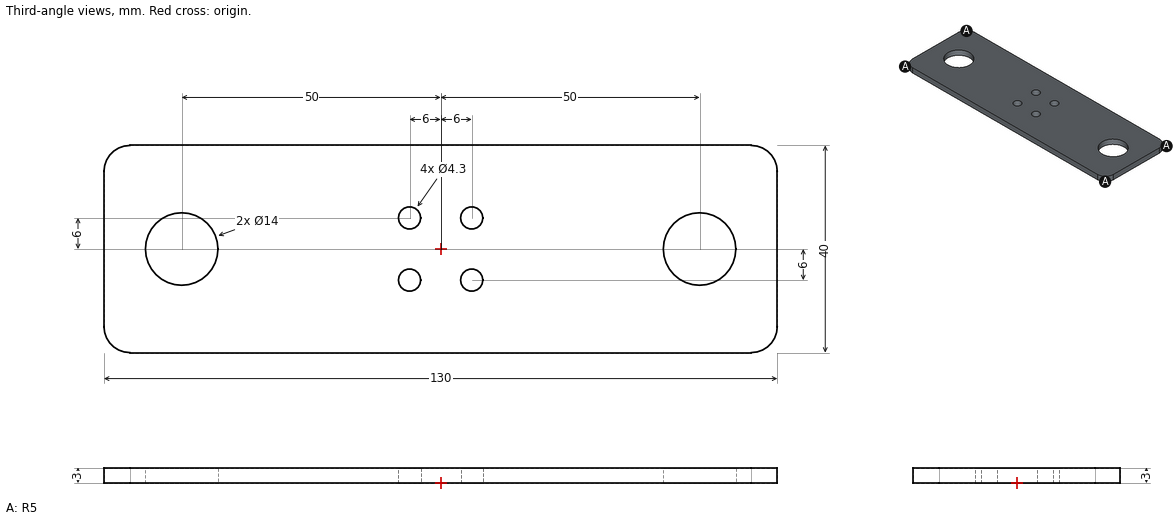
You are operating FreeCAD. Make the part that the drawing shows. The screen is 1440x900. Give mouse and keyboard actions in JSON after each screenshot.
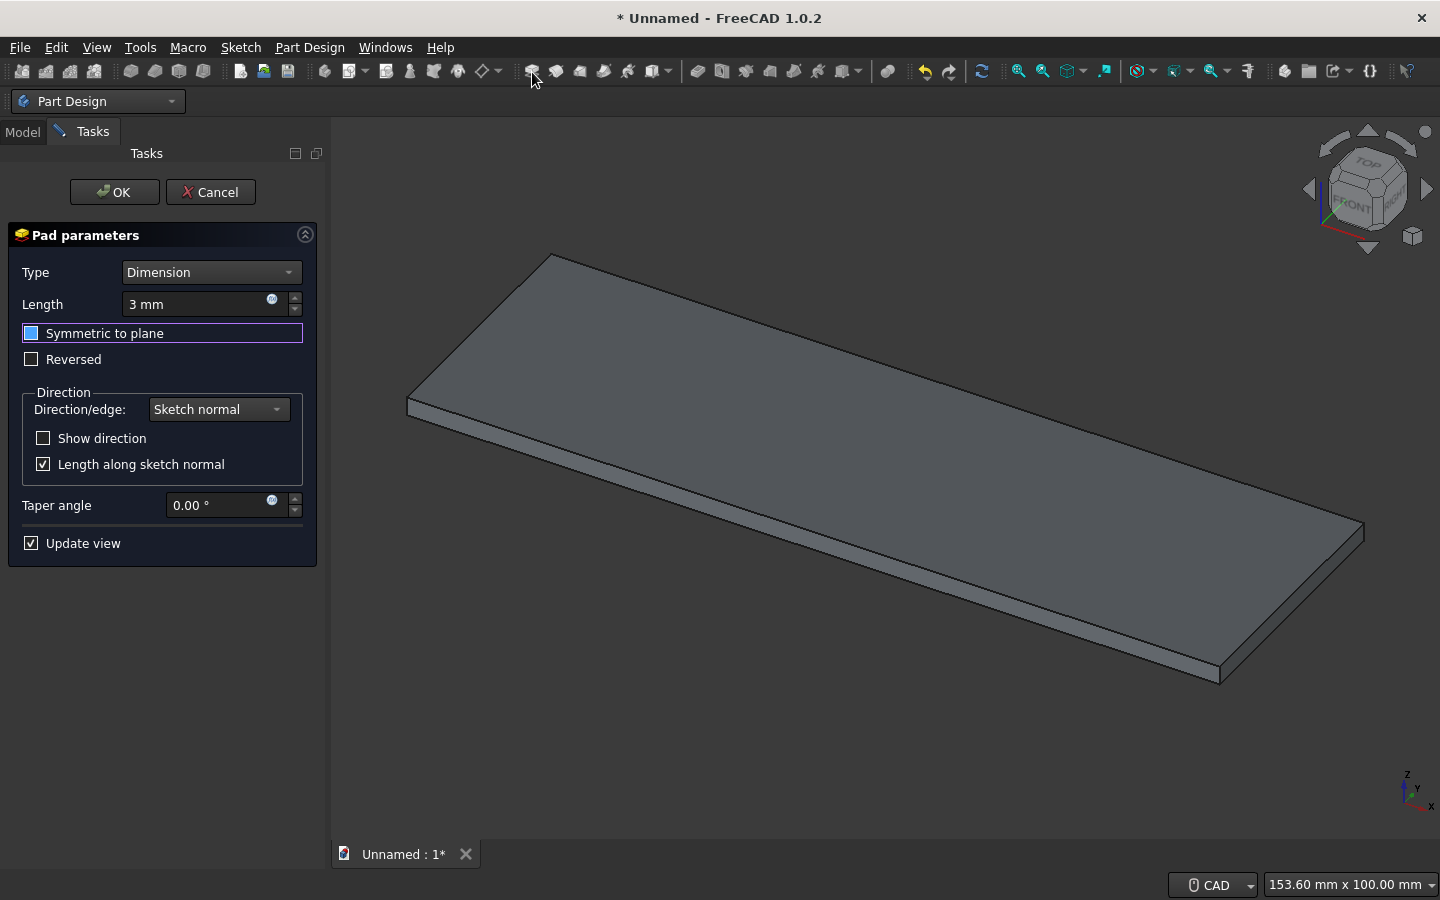
{"action": "left_click", "coordinate": [115, 192]}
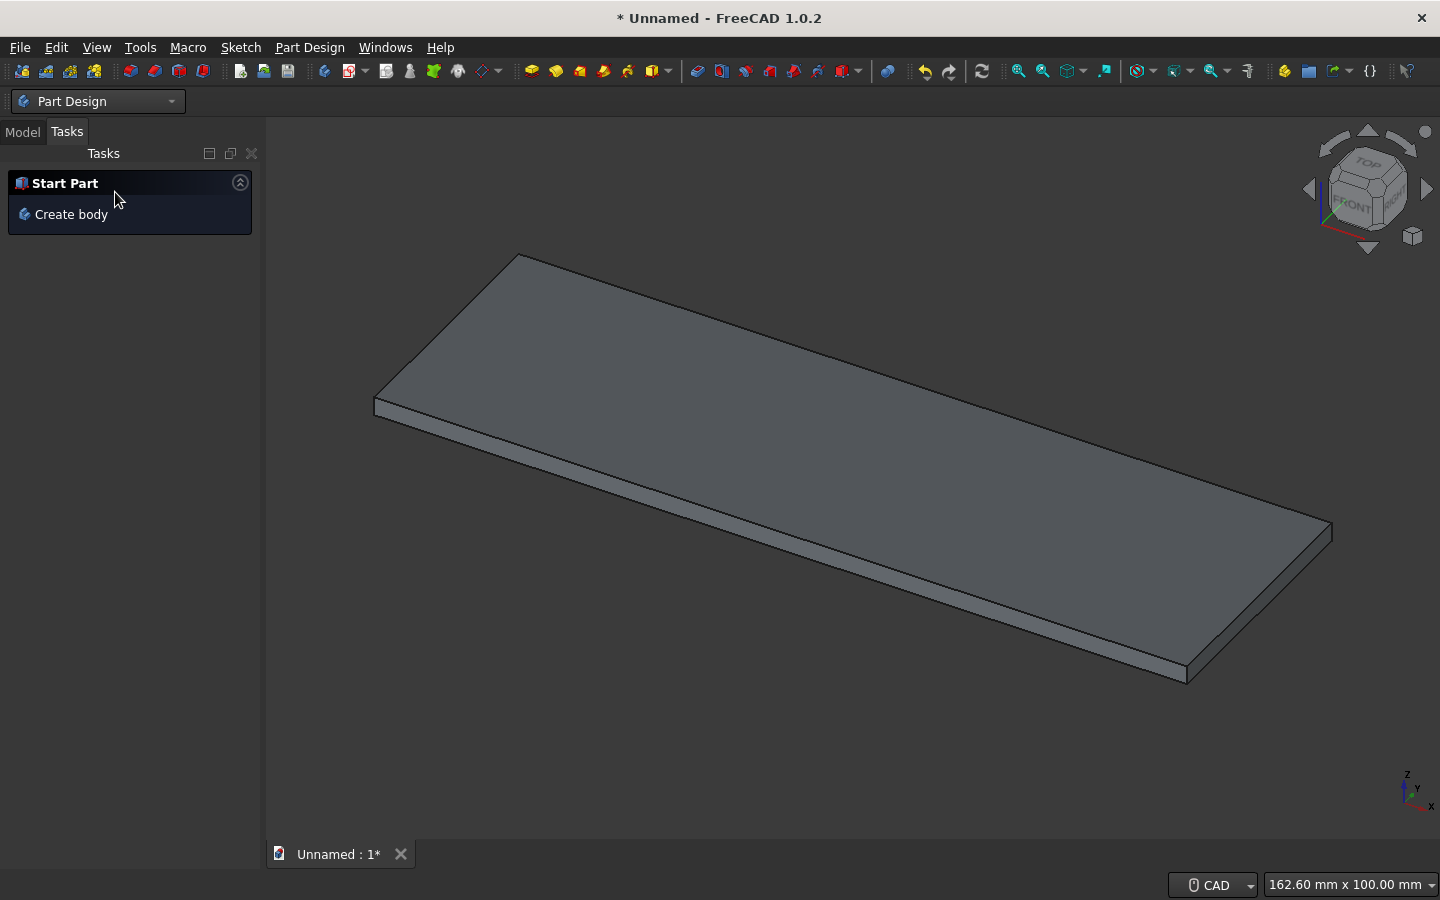
{"action": "left_click", "coordinate": [1085, 536]}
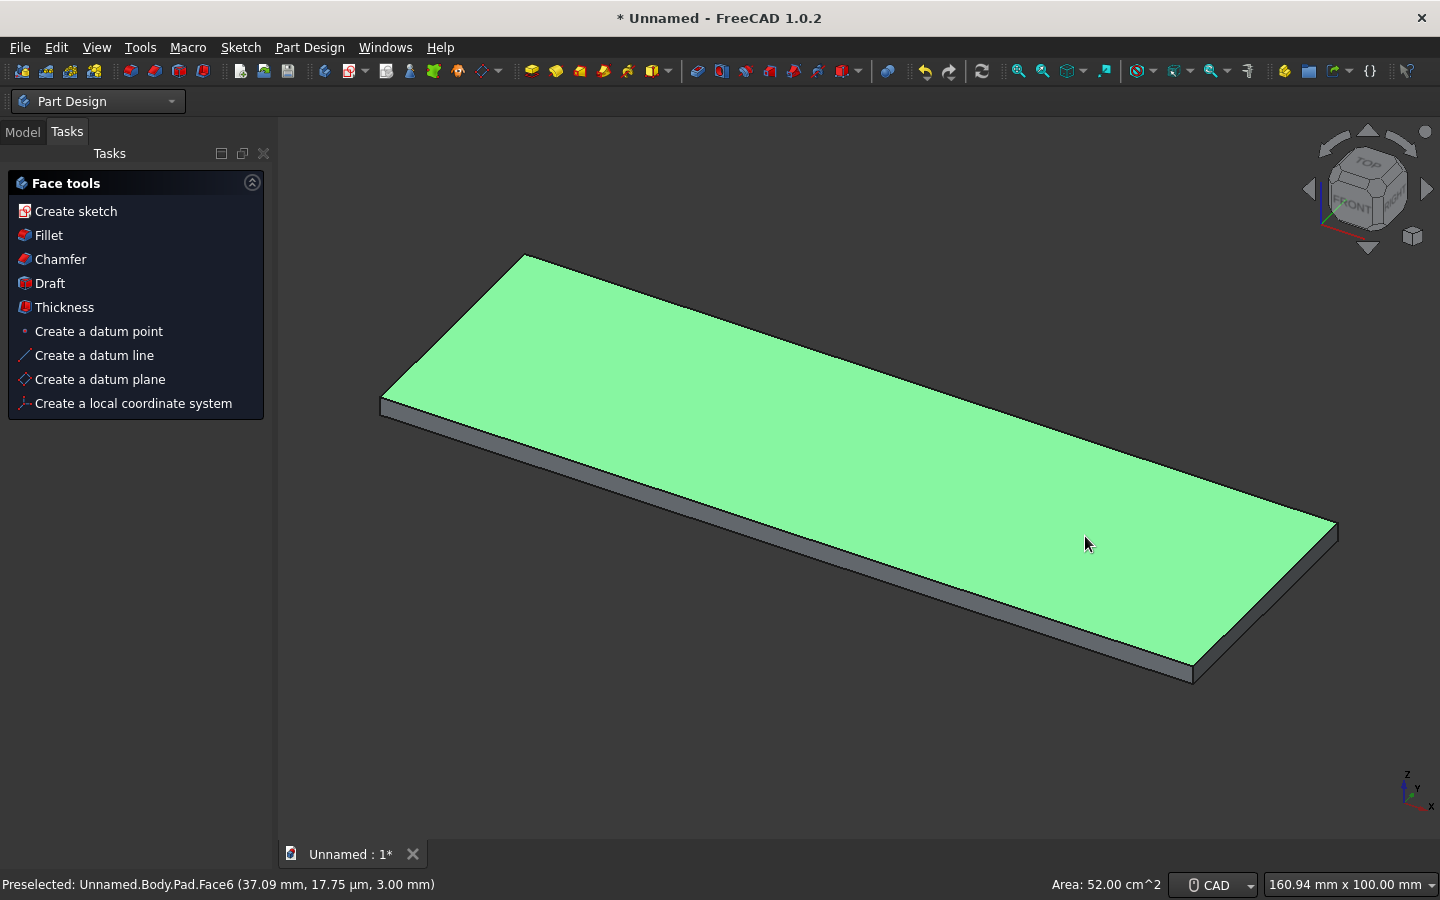
{"action": "left_click", "coordinate": [350, 72]}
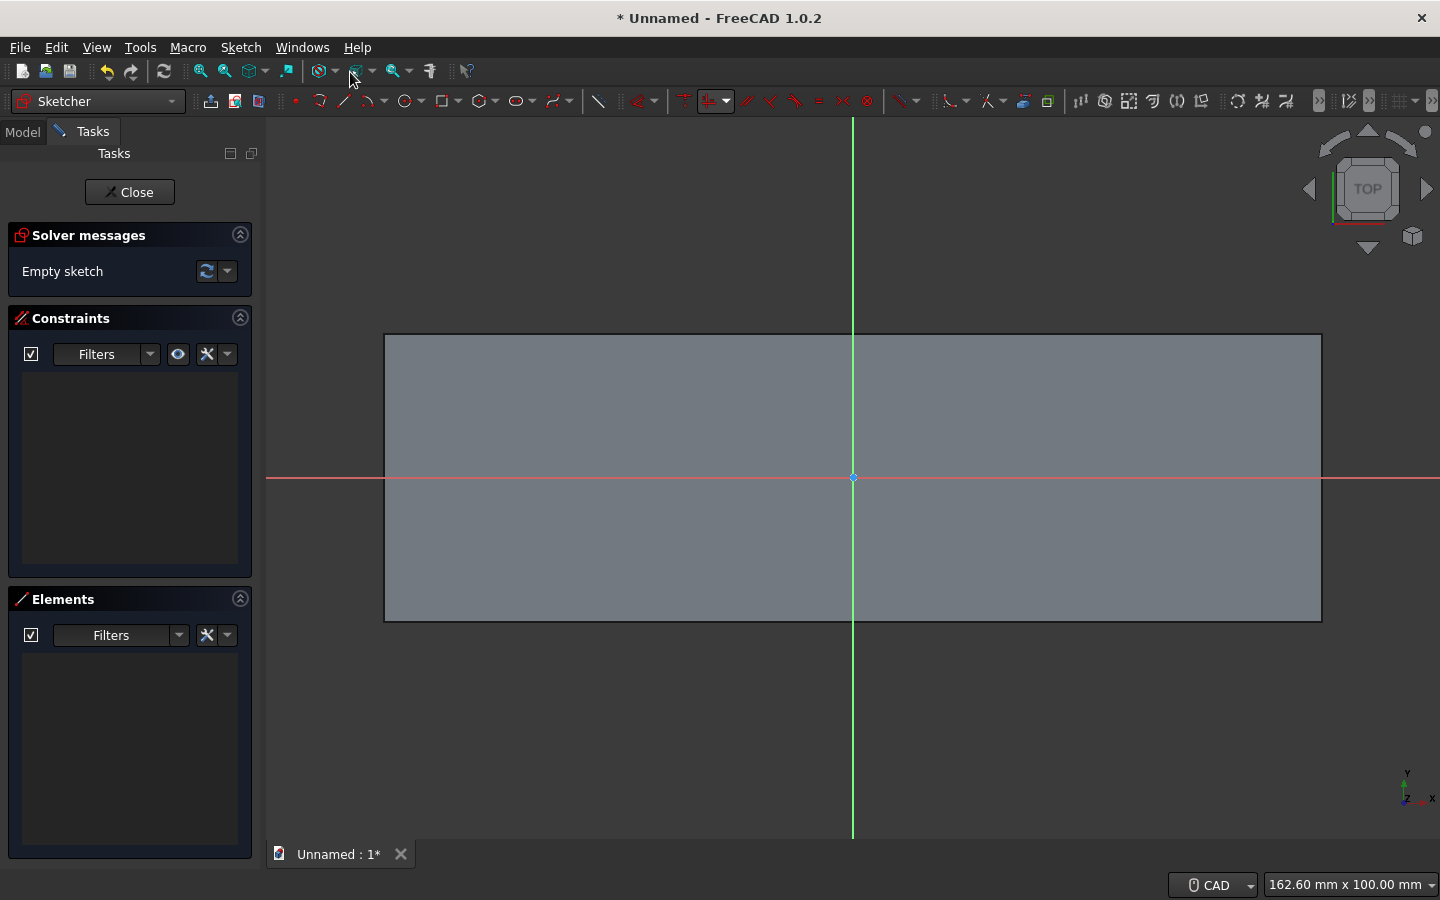
{"action": "scroll", "coordinate": [475, 478], "scroll_direction": "down", "scroll_amount": 1}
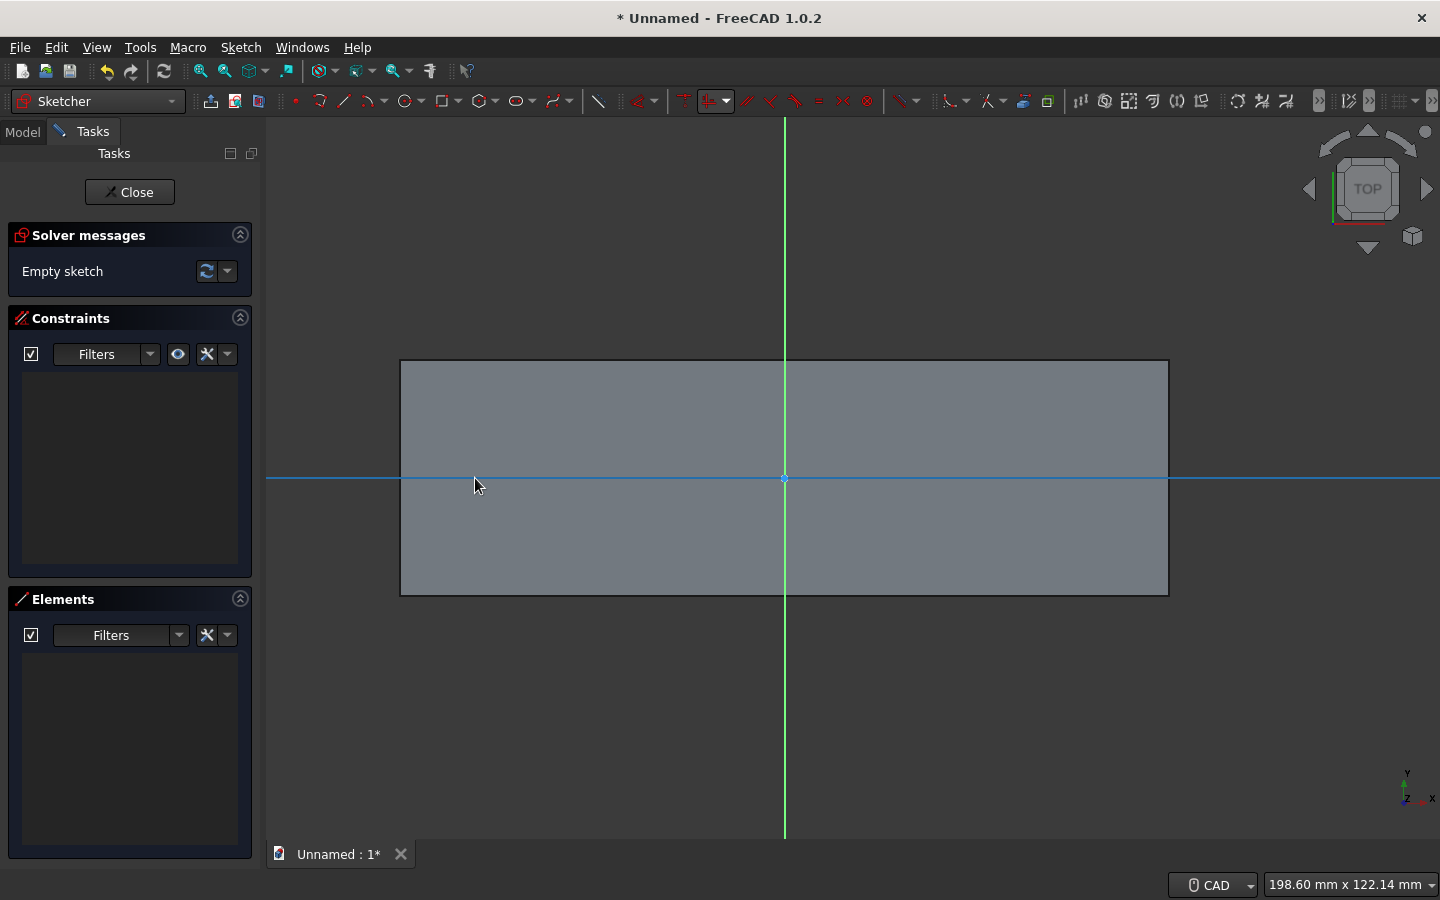
{"action": "key", "text": "g c"}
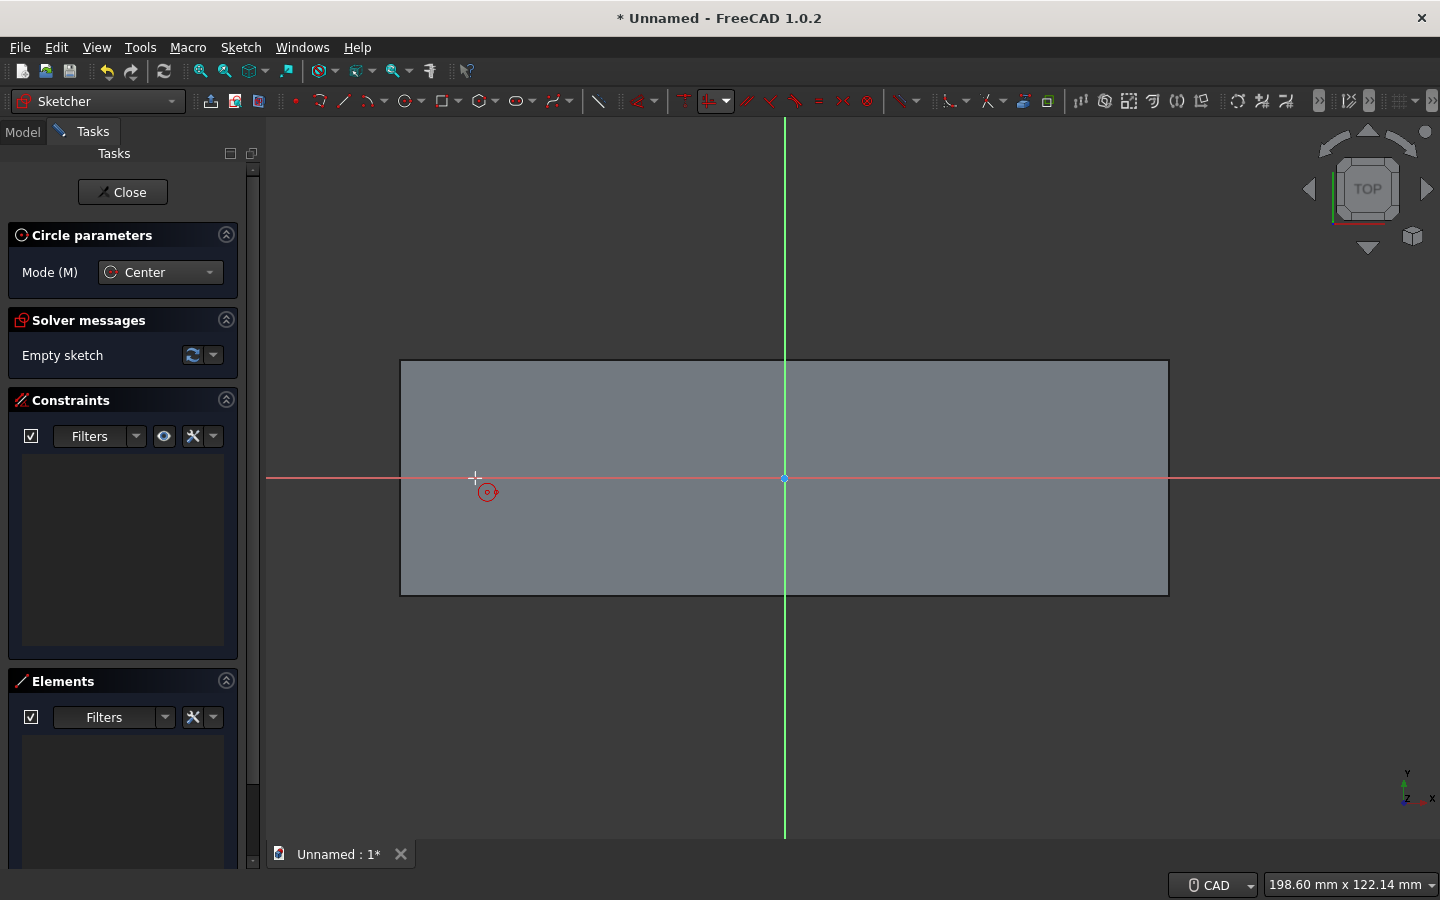
{"action": "left_click", "coordinate": [489, 478]}
{"action": "left_click", "coordinate": [518, 449]}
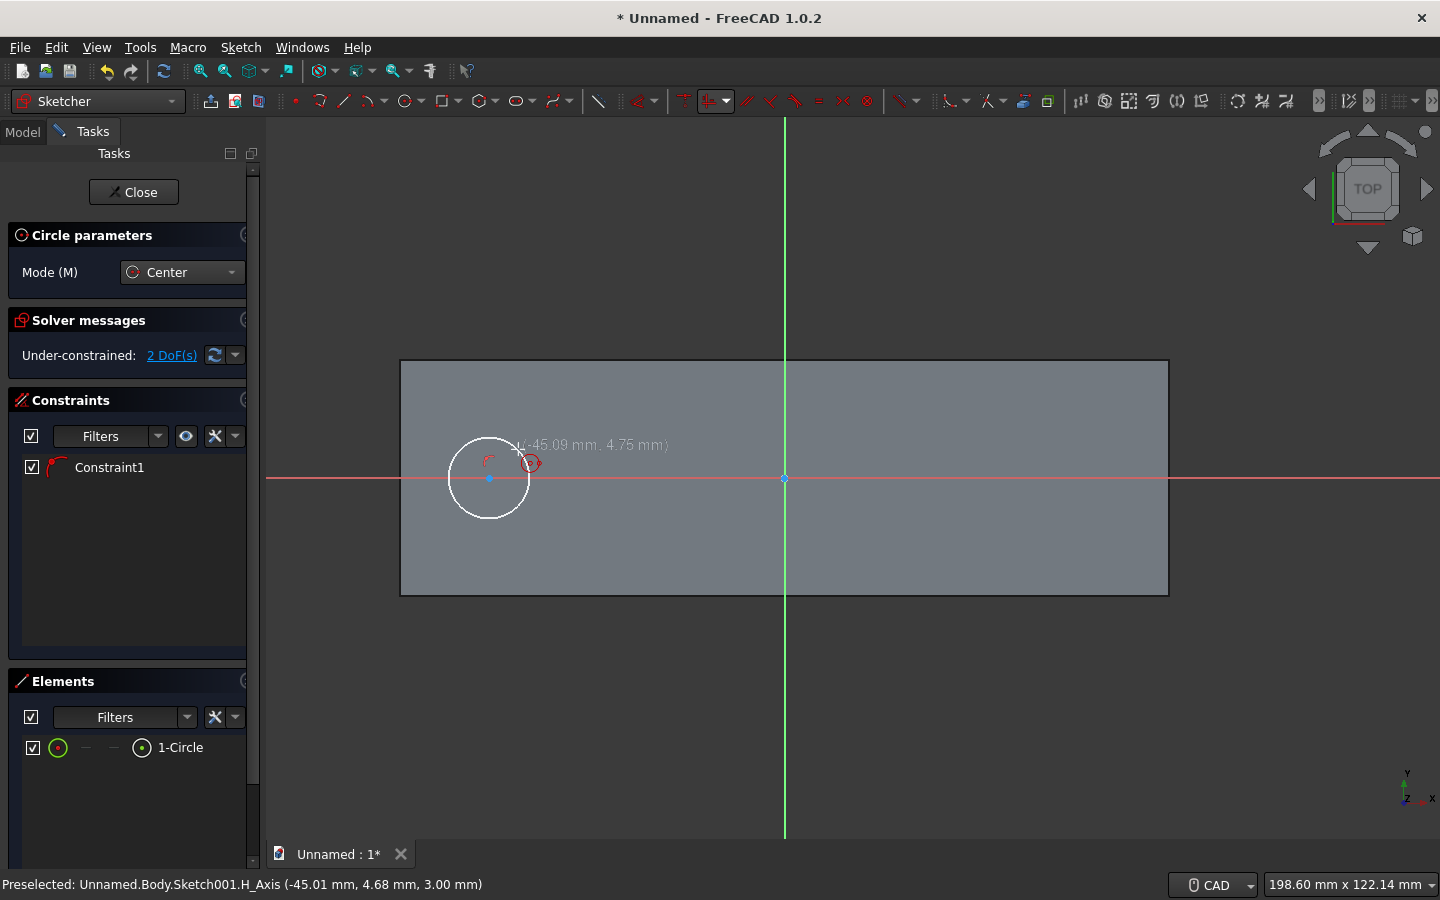
{"action": "left_click", "coordinate": [1080, 478]}
{"action": "left_click", "coordinate": [1109, 449]}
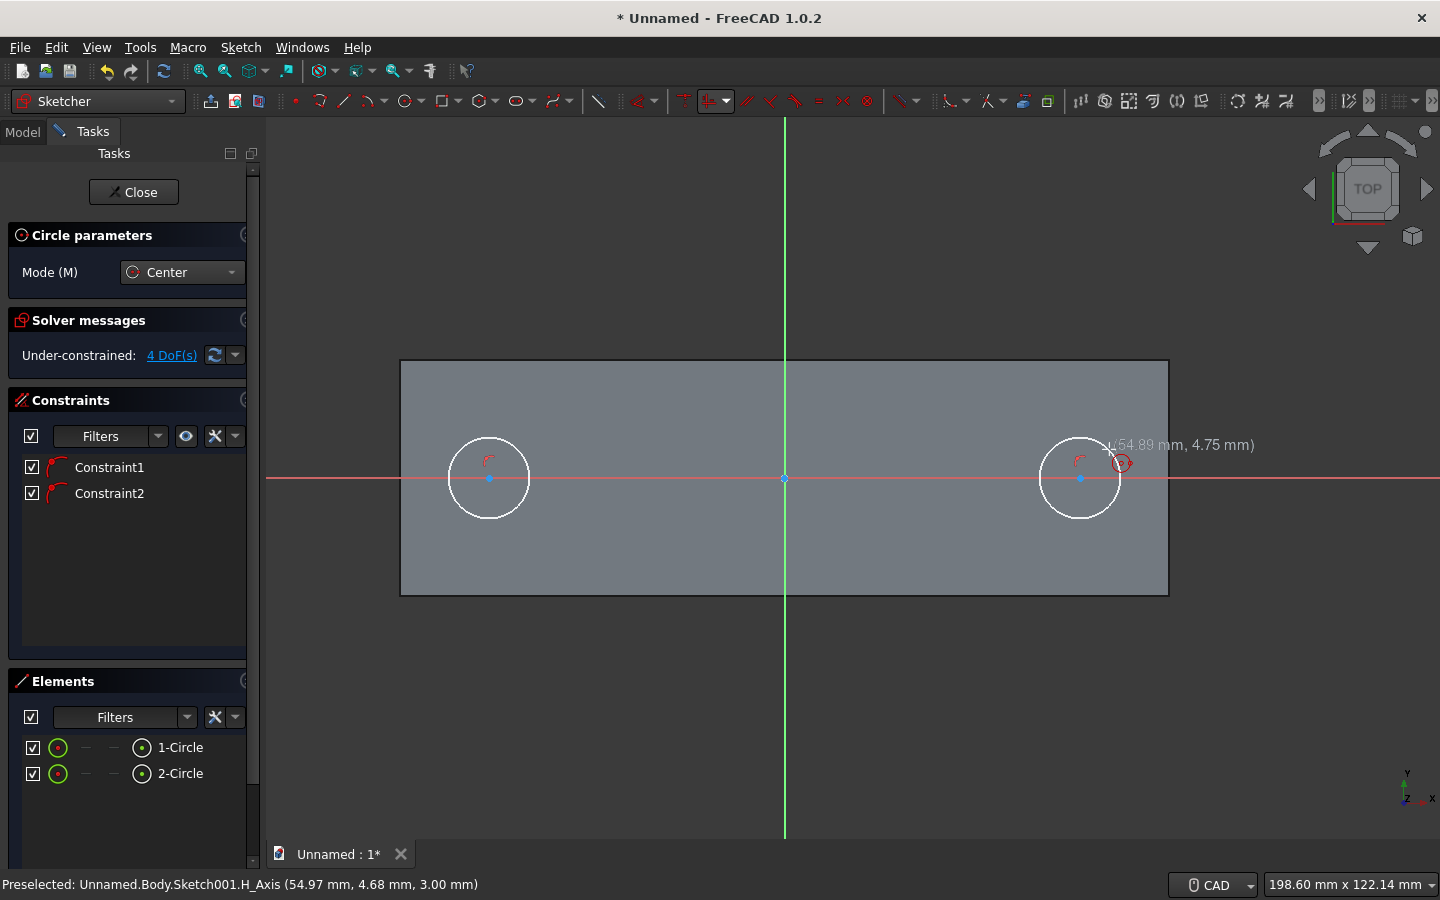
{"action": "scroll", "coordinate": [749, 443], "scroll_direction": "up", "scroll_amount": 3}